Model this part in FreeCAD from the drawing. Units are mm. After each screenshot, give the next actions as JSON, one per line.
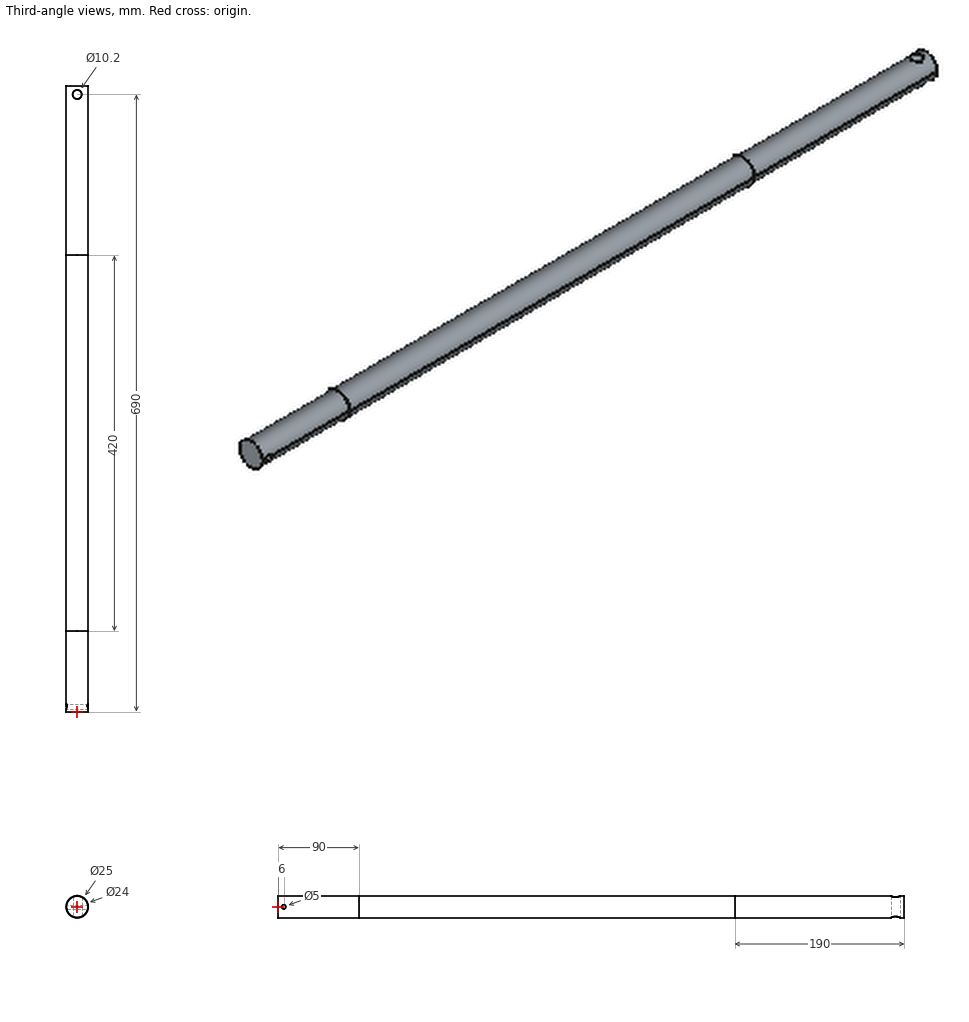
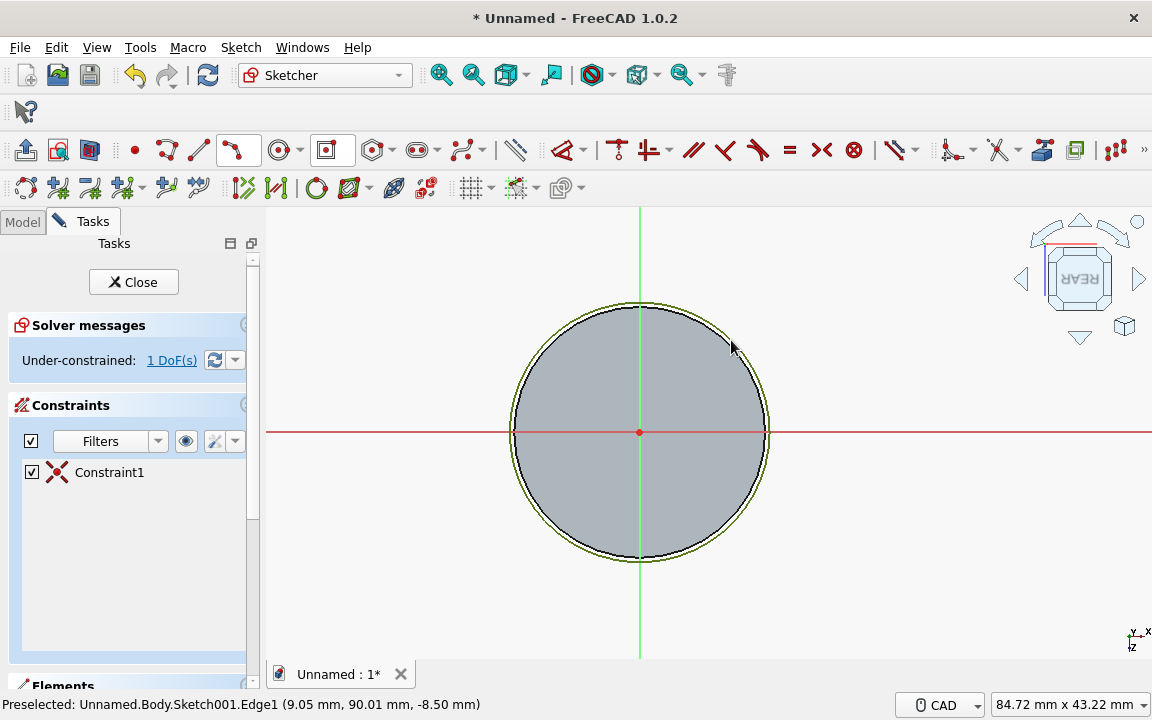
{"action": "left_click", "coordinate": [586, 150]}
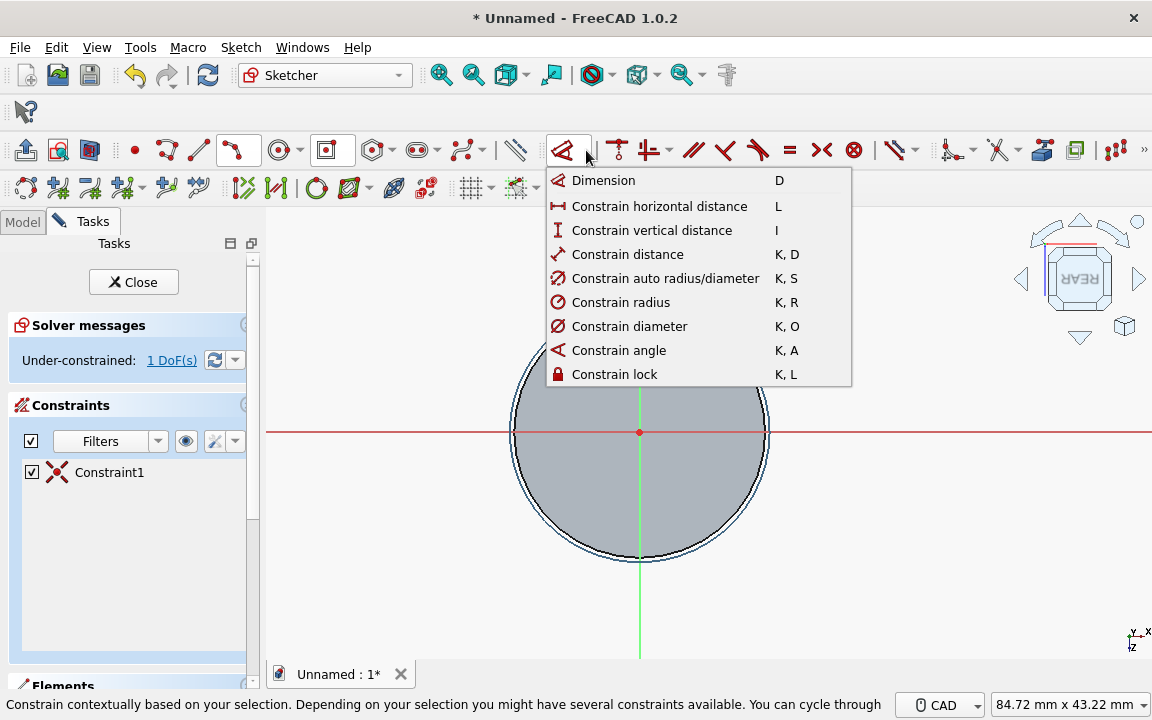
{"action": "left_click", "coordinate": [699, 326]}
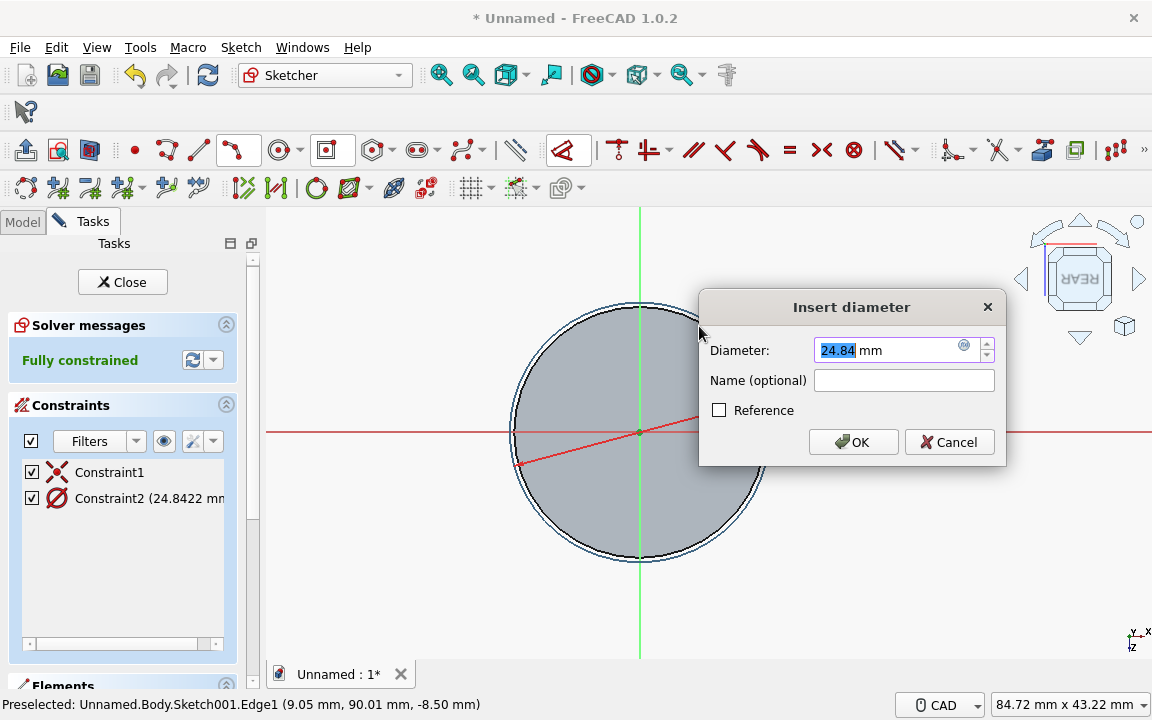
{"action": "type", "text": "25"}
{"action": "key", "text": "Return"}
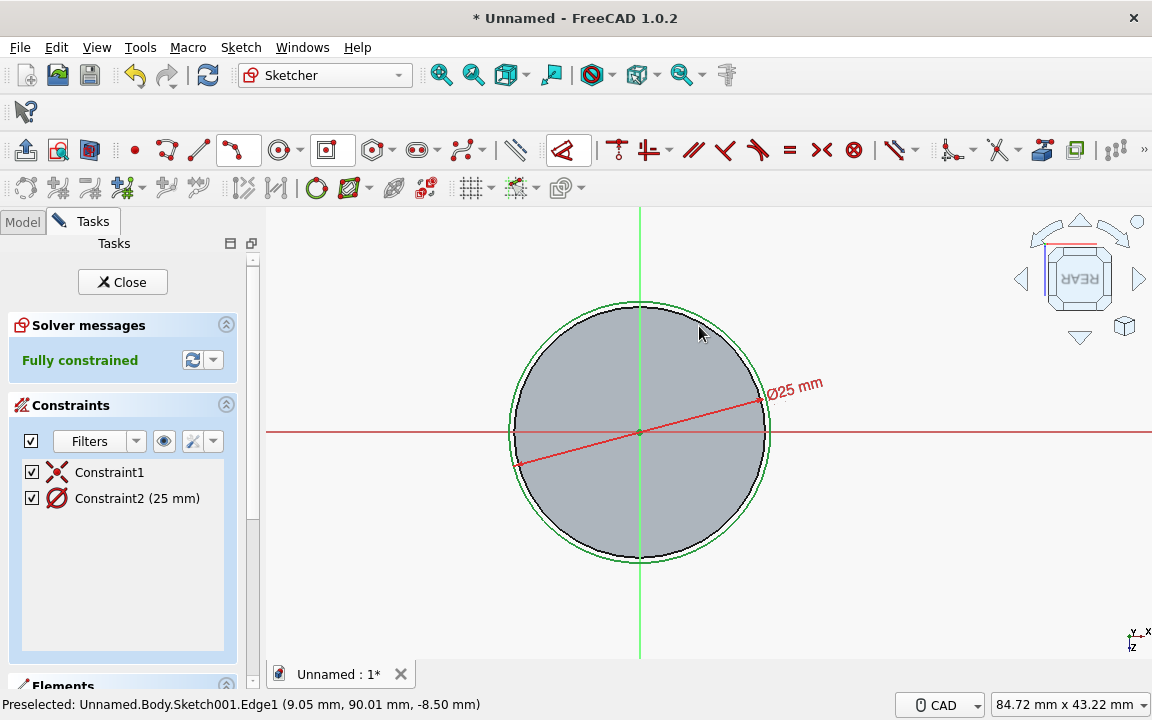
{"action": "left_click", "coordinate": [123, 282]}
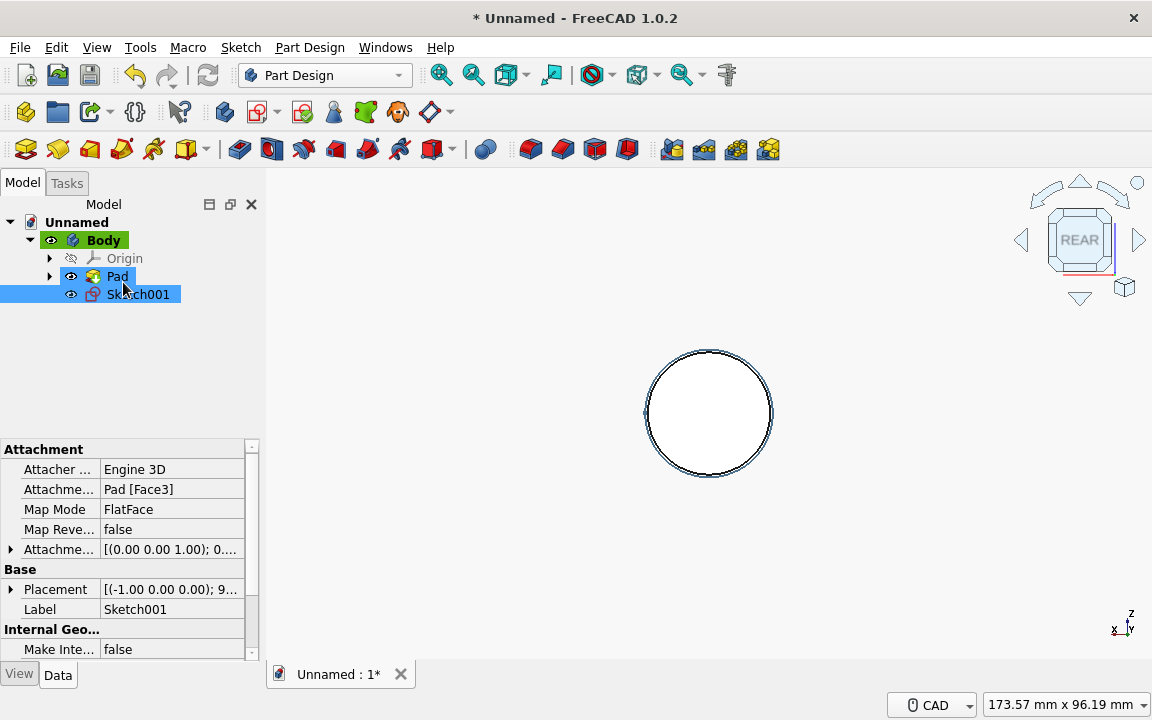
{"action": "left_click", "coordinate": [26, 150]}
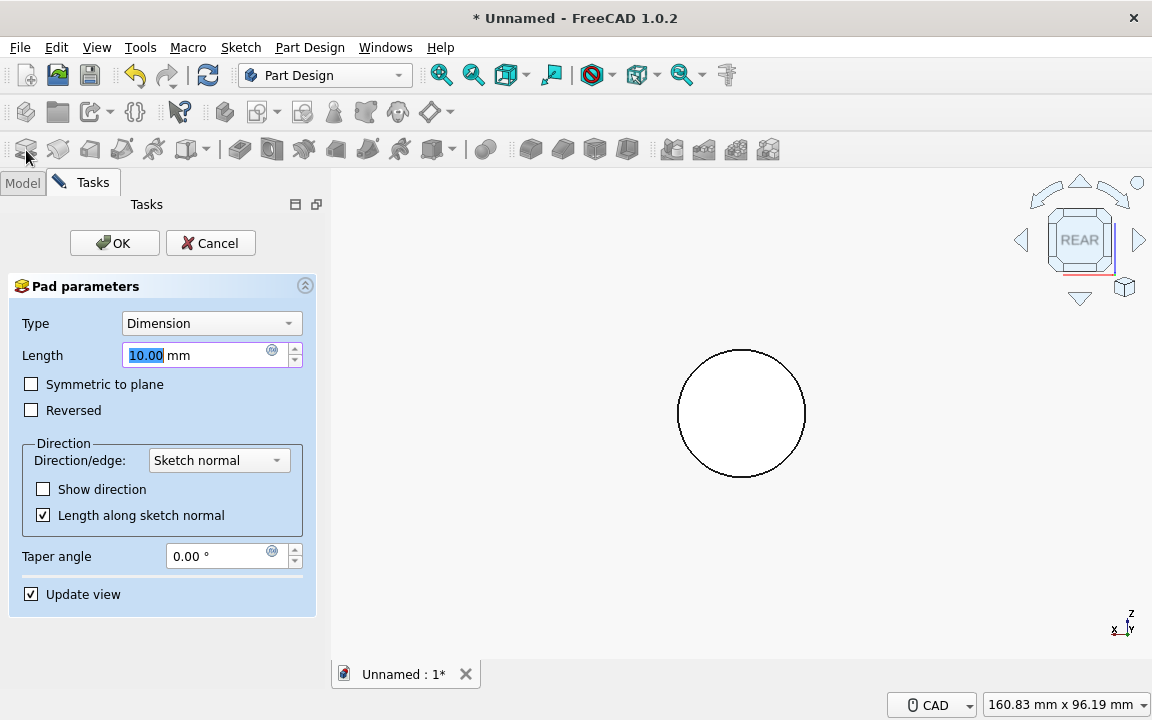
{"action": "type", "text": "420"}
{"action": "key", "text": "Tab"}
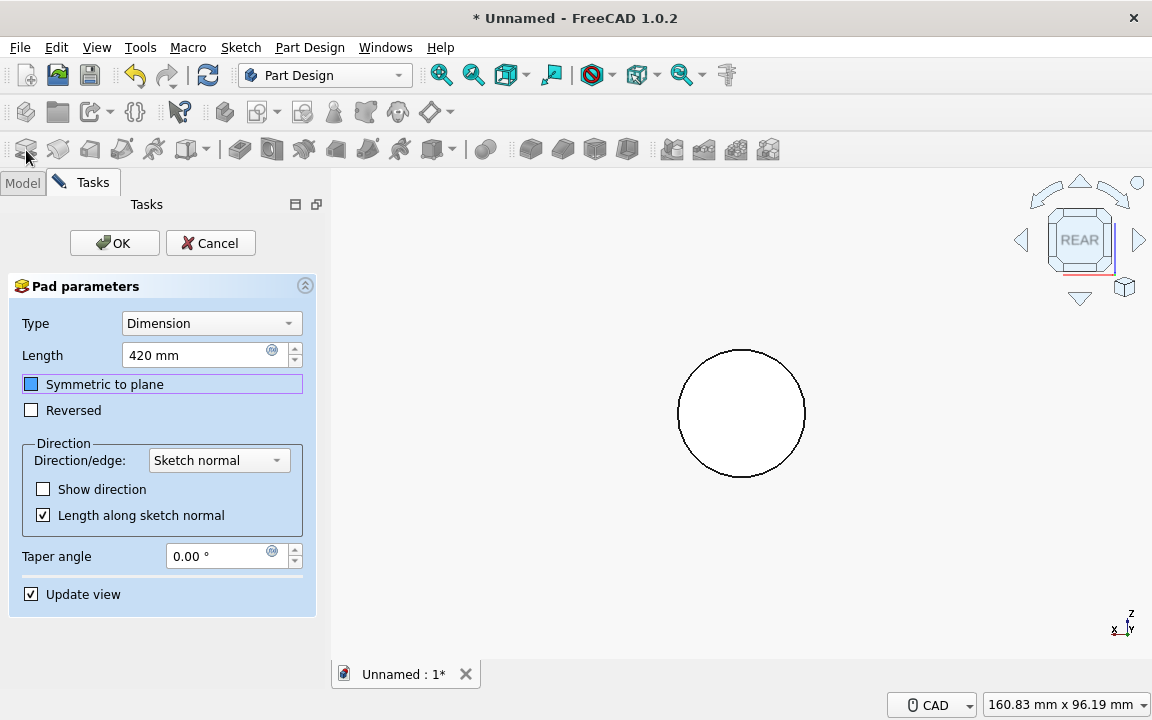
{"action": "left_click", "coordinate": [115, 243]}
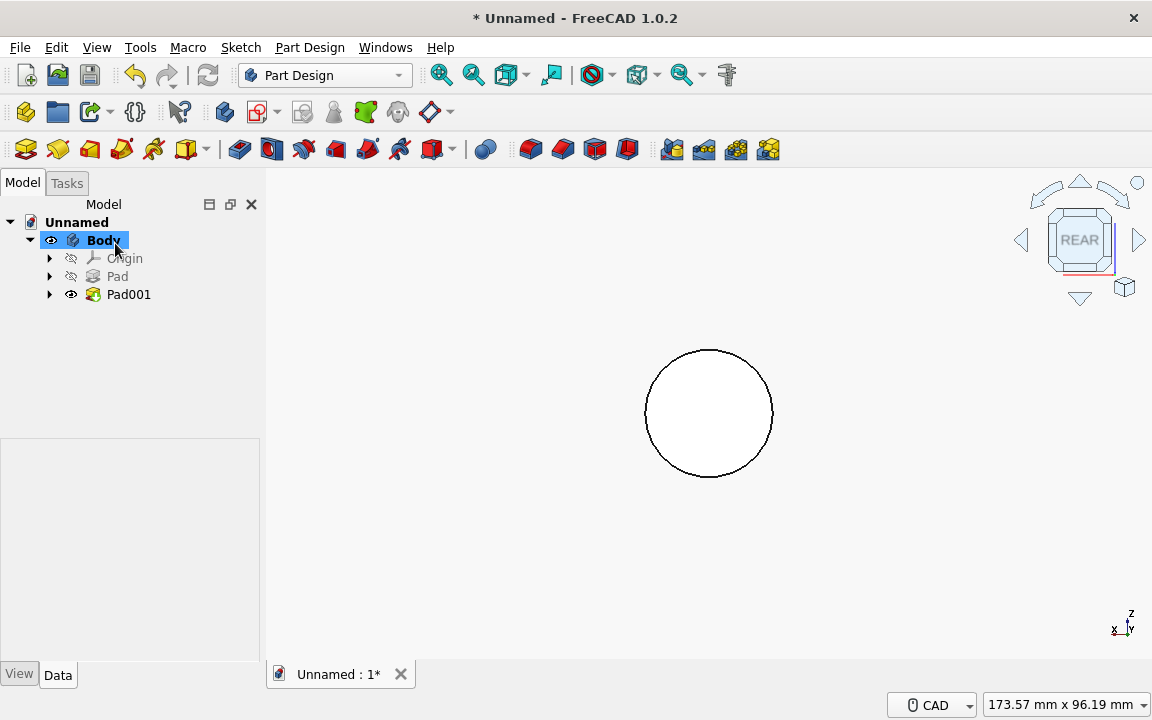
{"action": "left_click", "coordinate": [442, 76]}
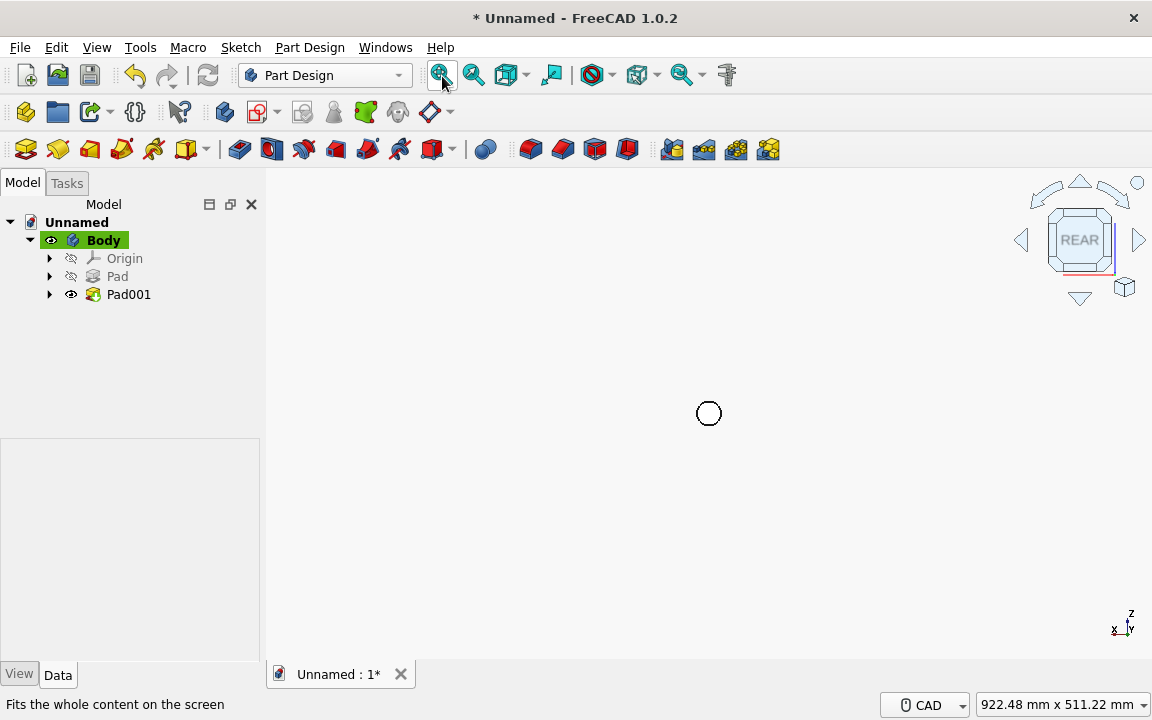
{"action": "left_click", "coordinate": [709, 412]}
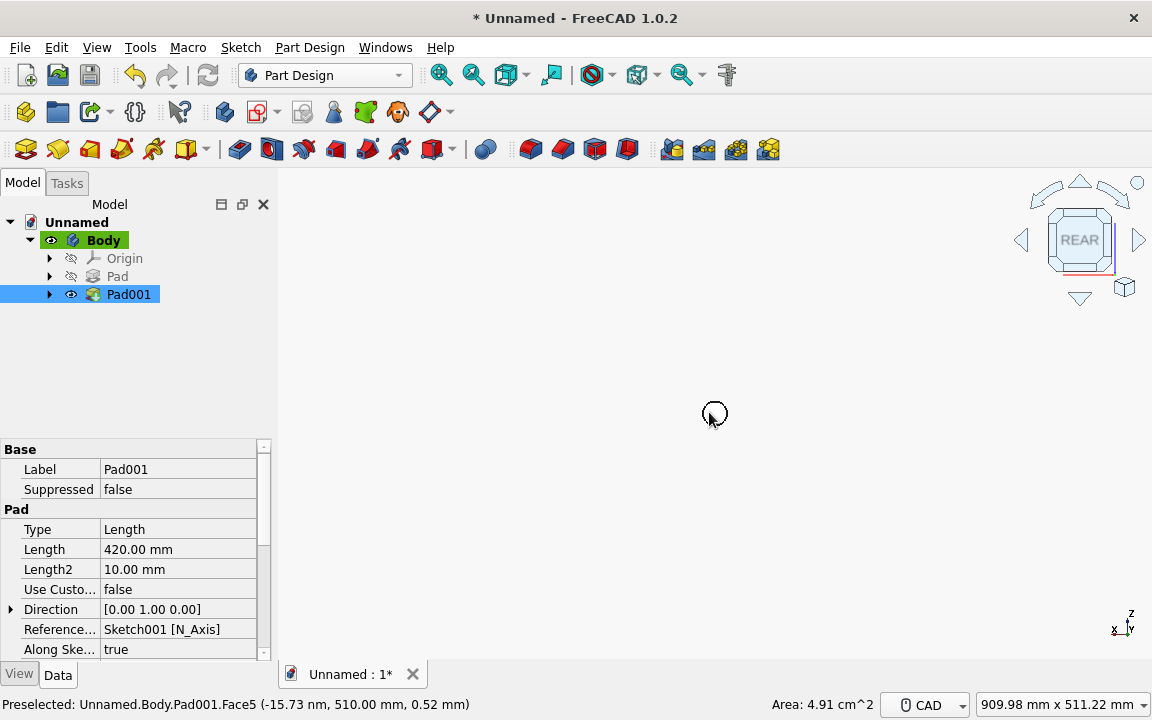
{"action": "left_click", "coordinate": [258, 112]}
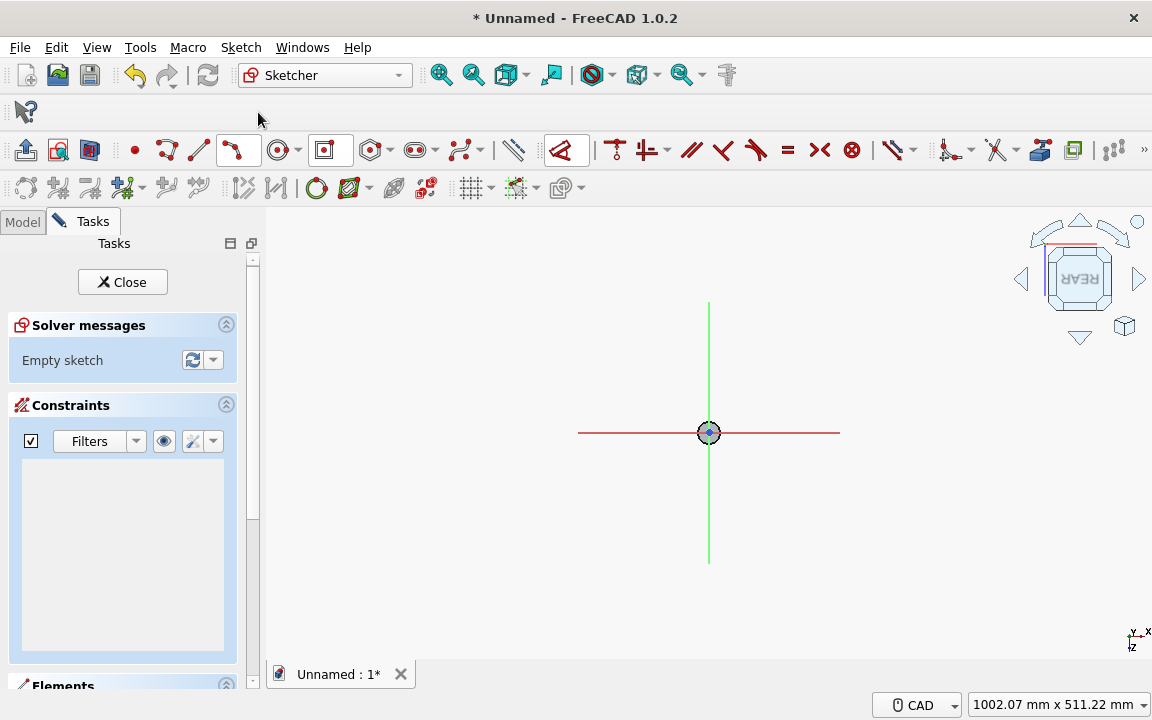
{"action": "scroll", "coordinate": [714, 433], "scroll_direction": "up", "scroll_amount": 13}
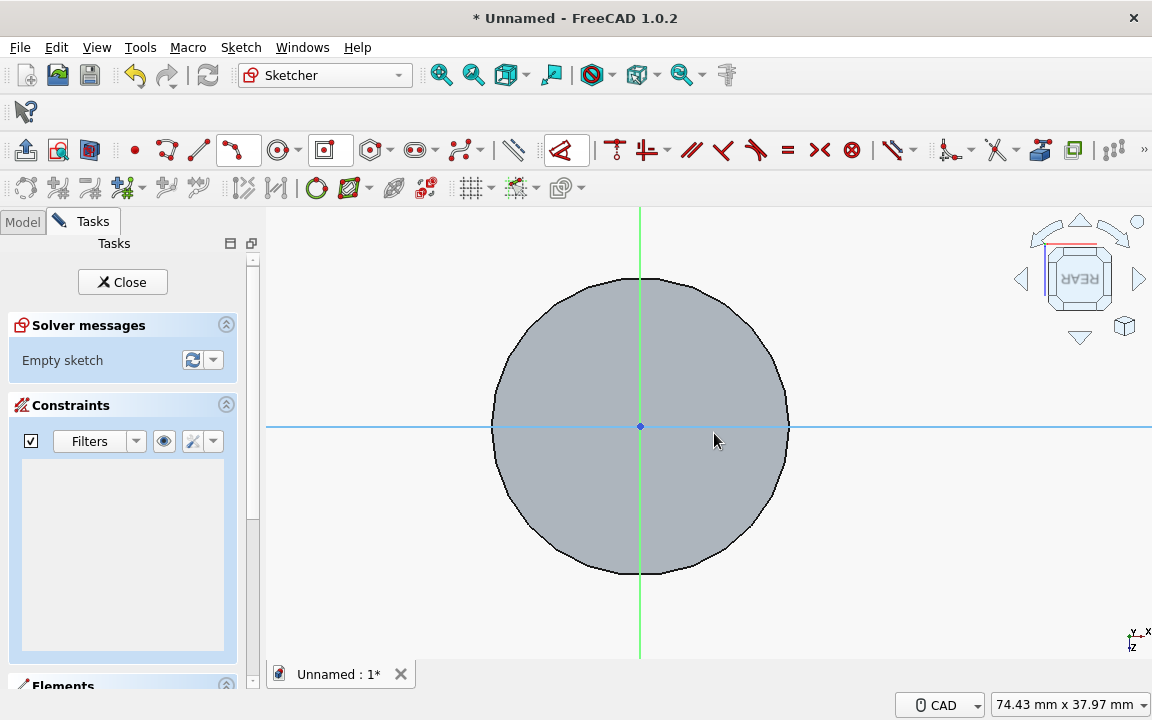
{"action": "left_click", "coordinate": [278, 150]}